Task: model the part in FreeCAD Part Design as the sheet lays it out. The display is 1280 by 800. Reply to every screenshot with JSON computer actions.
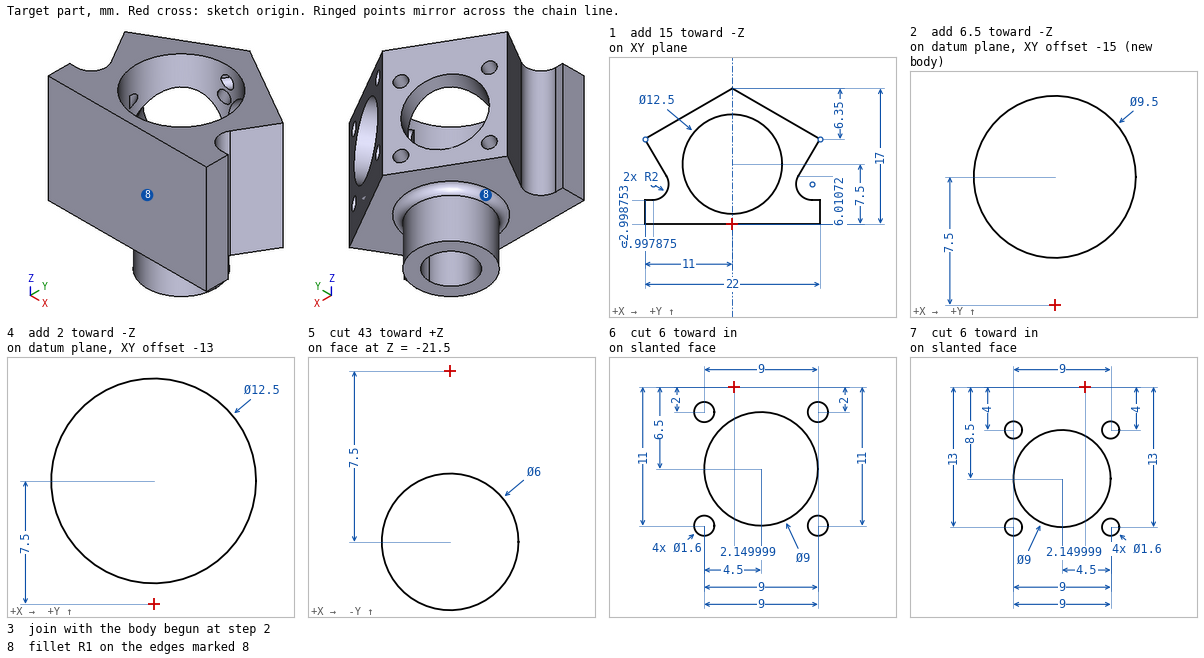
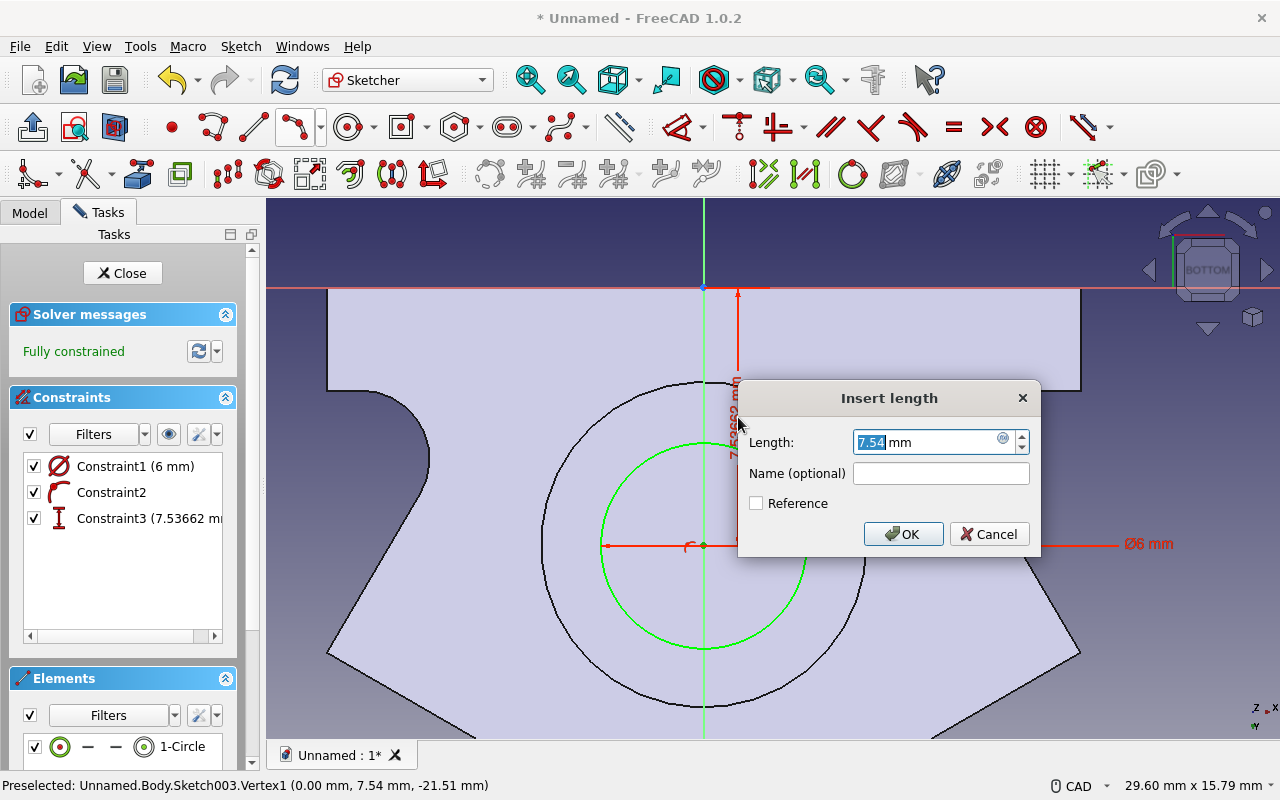
{"action": "type", "text": "7.5"}
{"action": "key", "text": "Return"}
{"action": "key", "text": "Escape"}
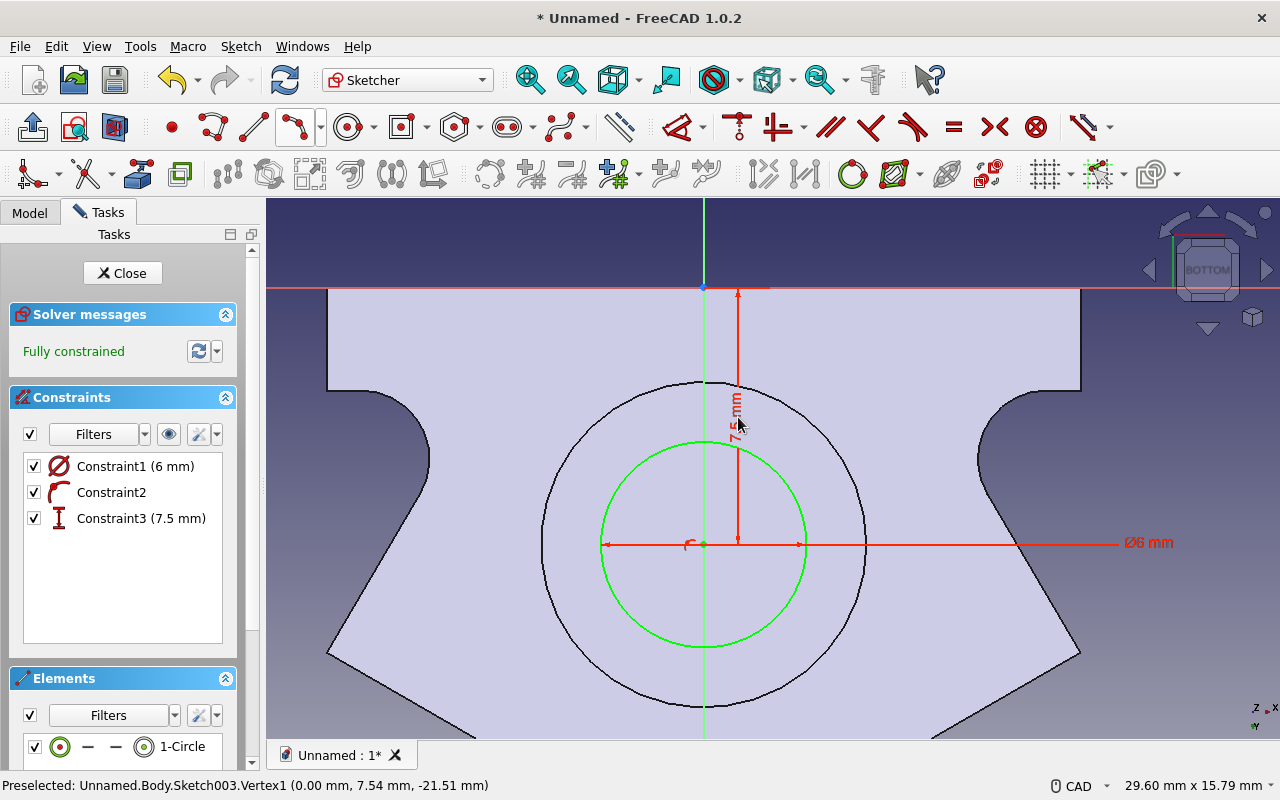
{"action": "left_click", "coordinate": [123, 273]}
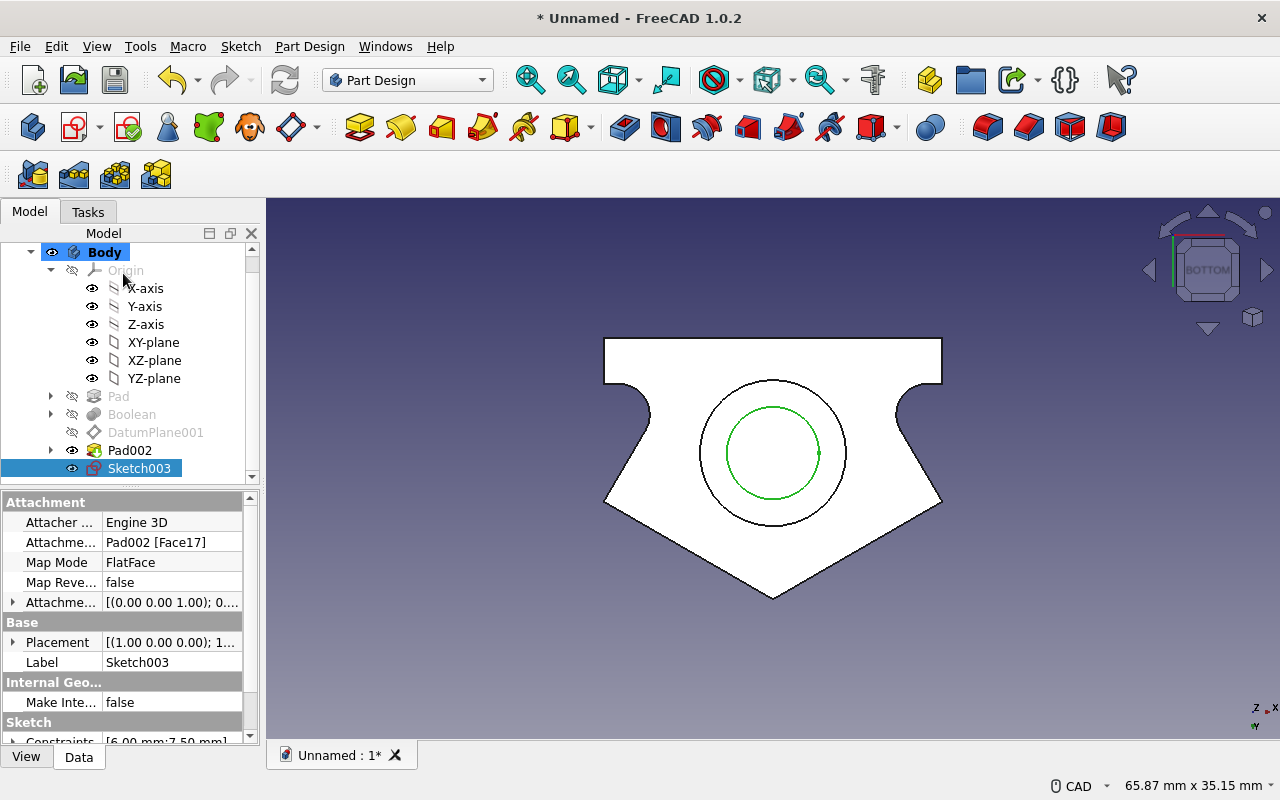
{"action": "left_click", "coordinate": [625, 128]}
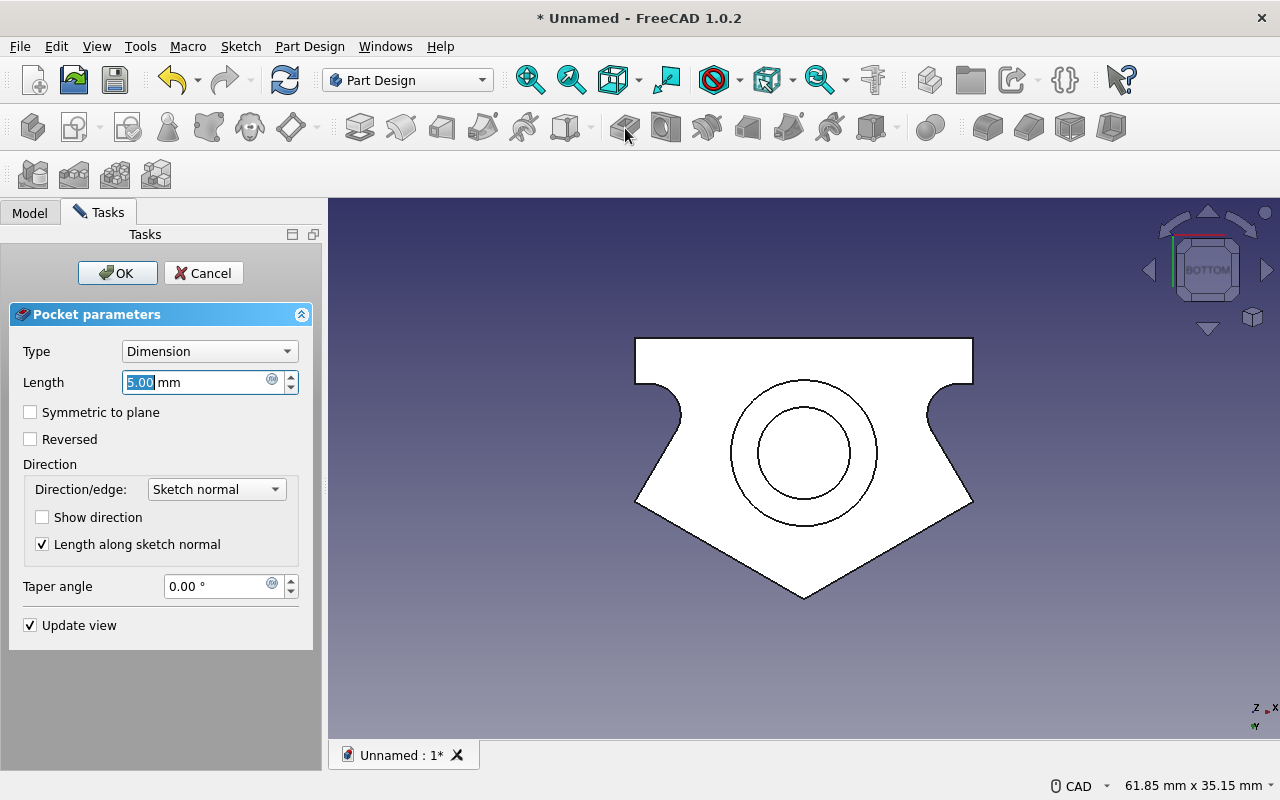
{"action": "type", "text": "43"}
{"action": "key", "text": "Tab"}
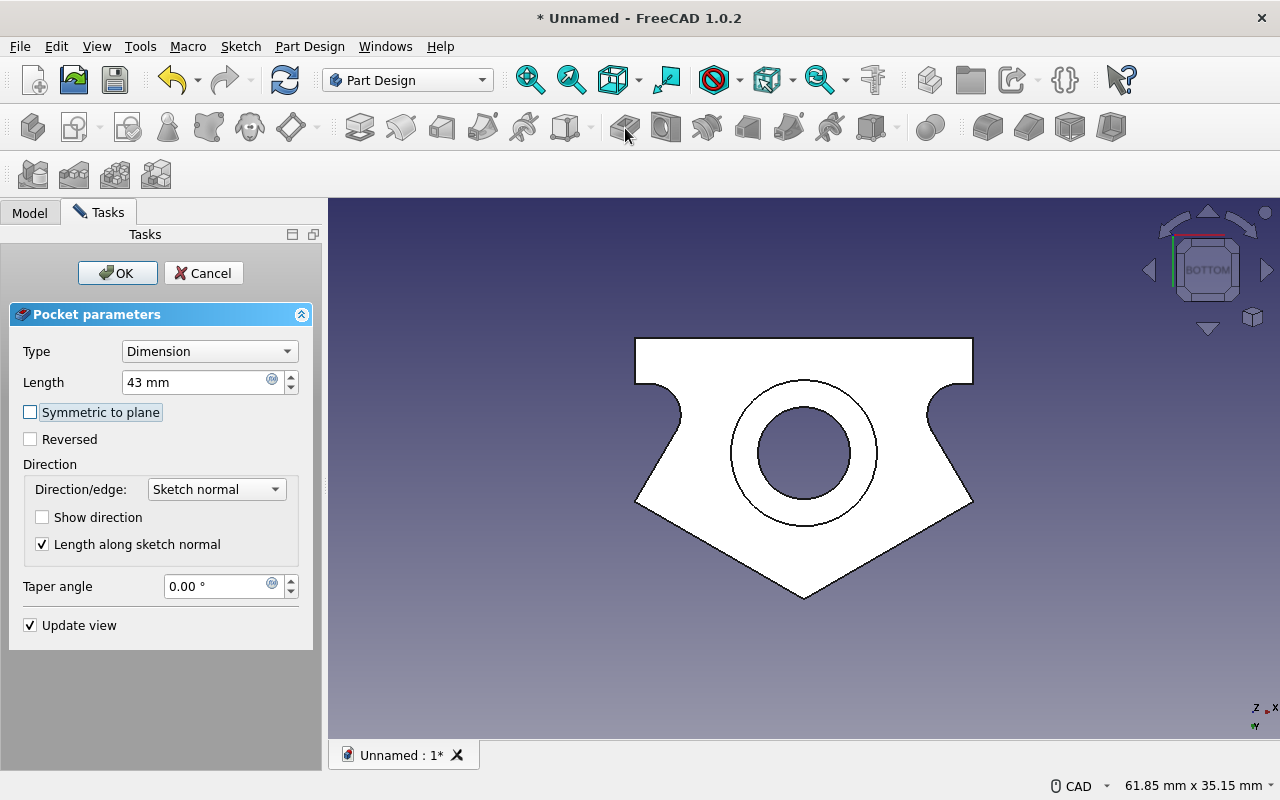
{"action": "left_click", "coordinate": [118, 273]}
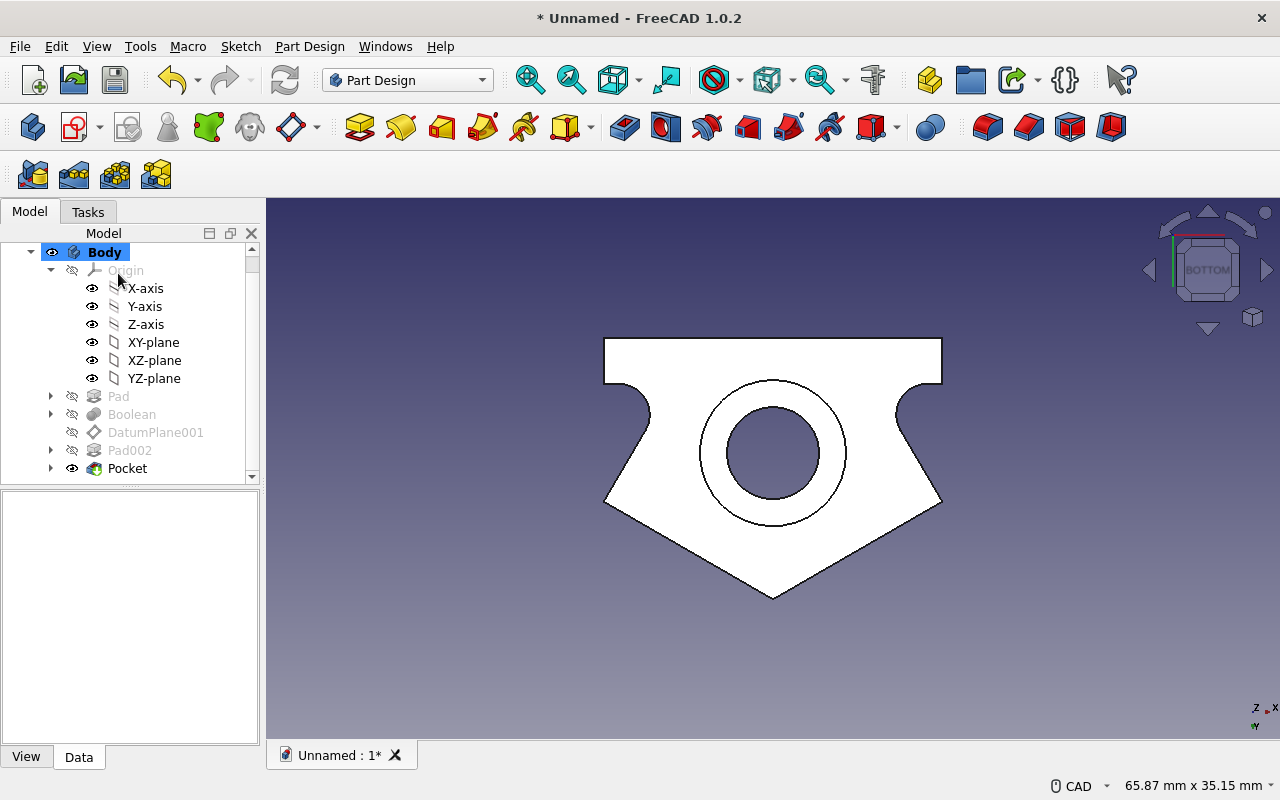
{"action": "key", "text": "4"}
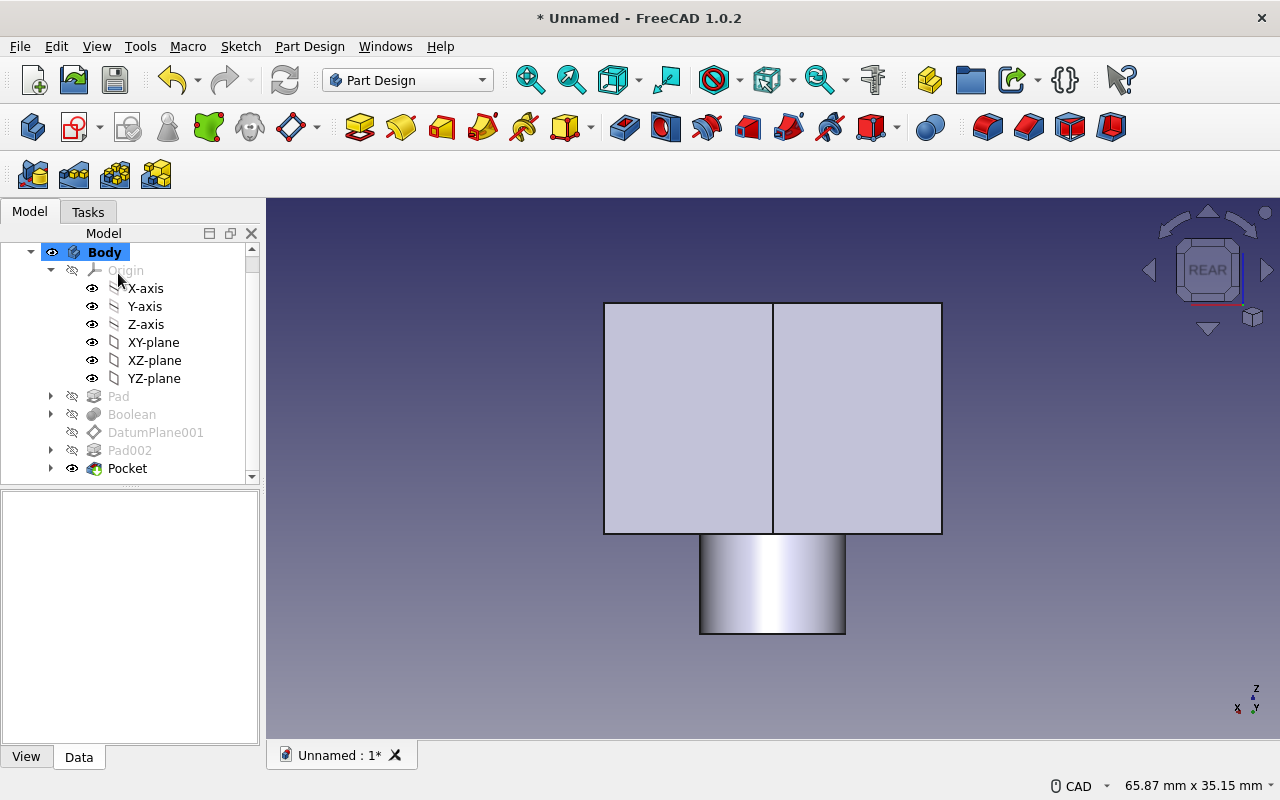
{"action": "left_click", "coordinate": [688, 417]}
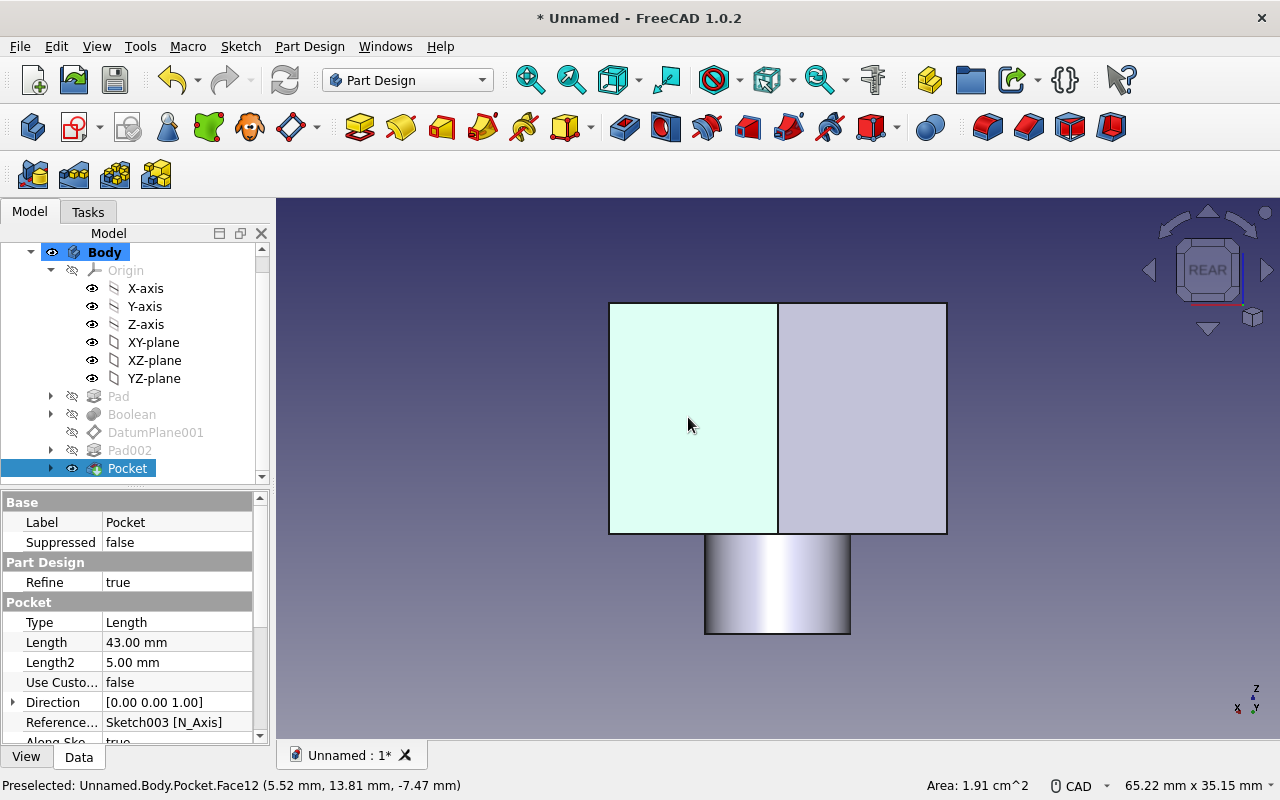
{"action": "left_click", "coordinate": [74, 128]}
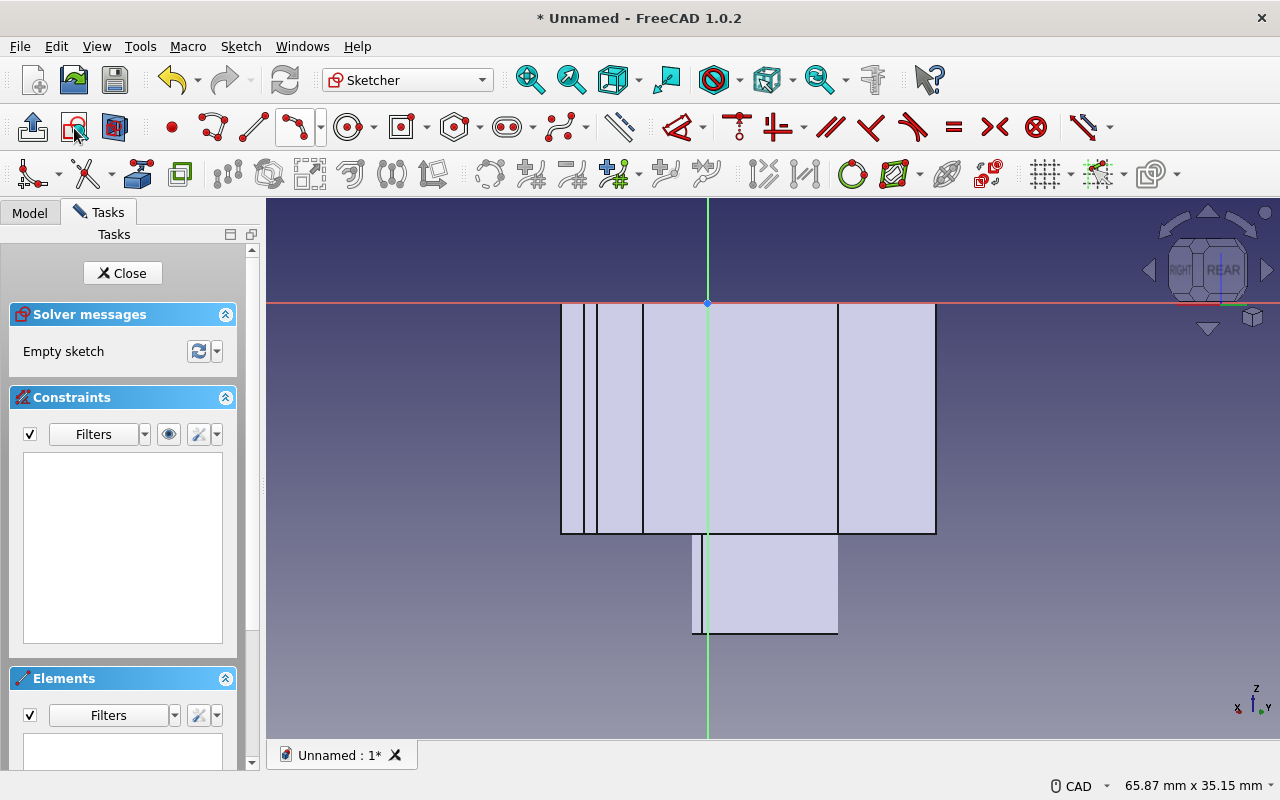
{"action": "left_click", "coordinate": [115, 128]}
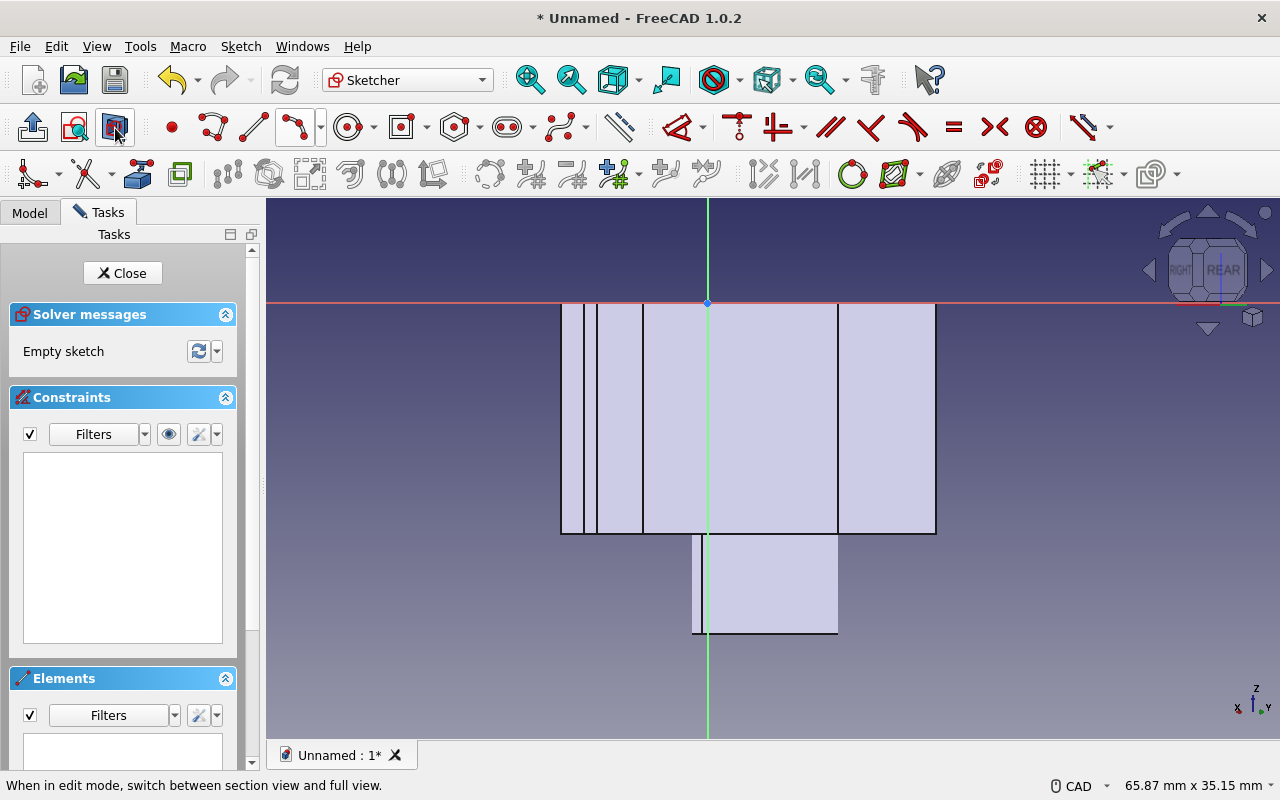
{"action": "scroll", "coordinate": [785, 303], "scroll_direction": "up", "scroll_amount": 3}